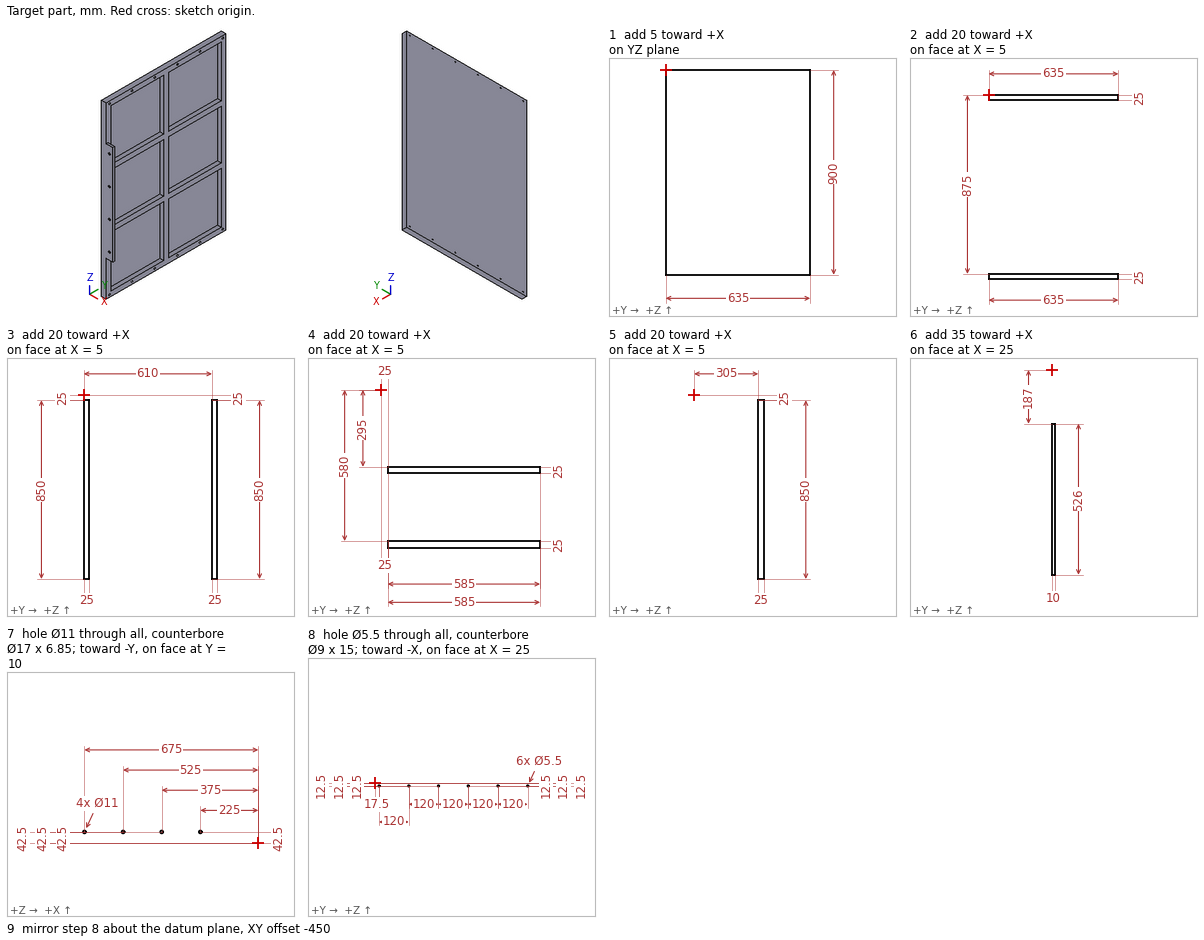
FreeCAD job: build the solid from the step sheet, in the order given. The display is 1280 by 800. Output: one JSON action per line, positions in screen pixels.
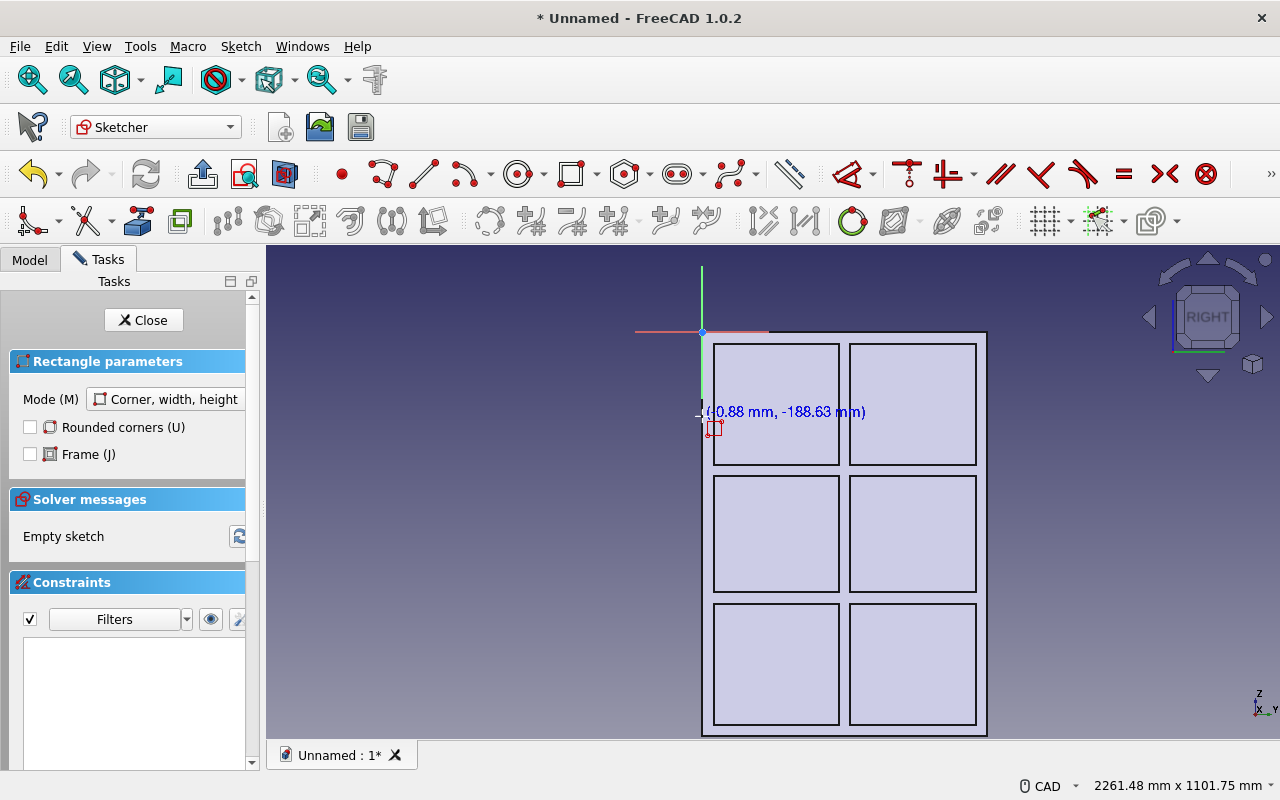
{"action": "left_click", "coordinate": [702, 416]}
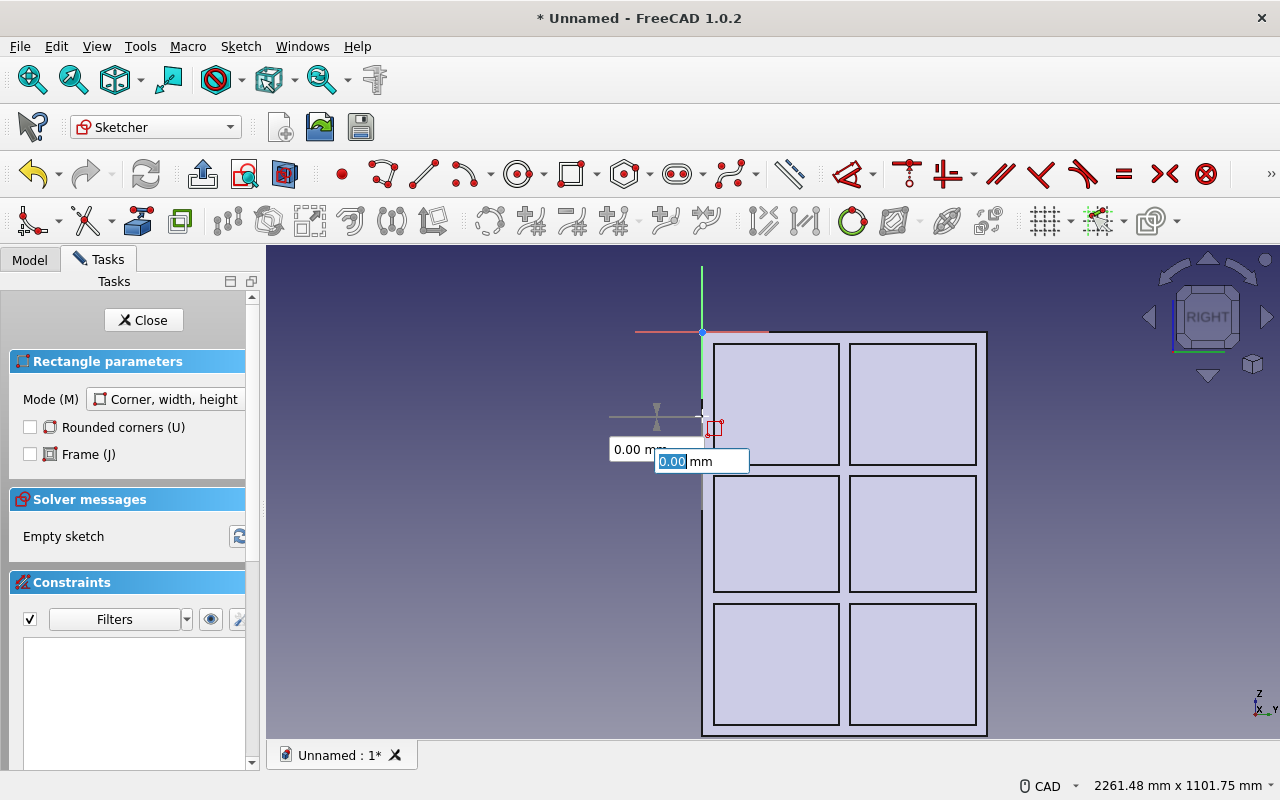
{"action": "scroll", "coordinate": [707, 652], "scroll_direction": "up", "scroll_amount": 7}
{"action": "mouse_move", "coordinate": [705, 650]}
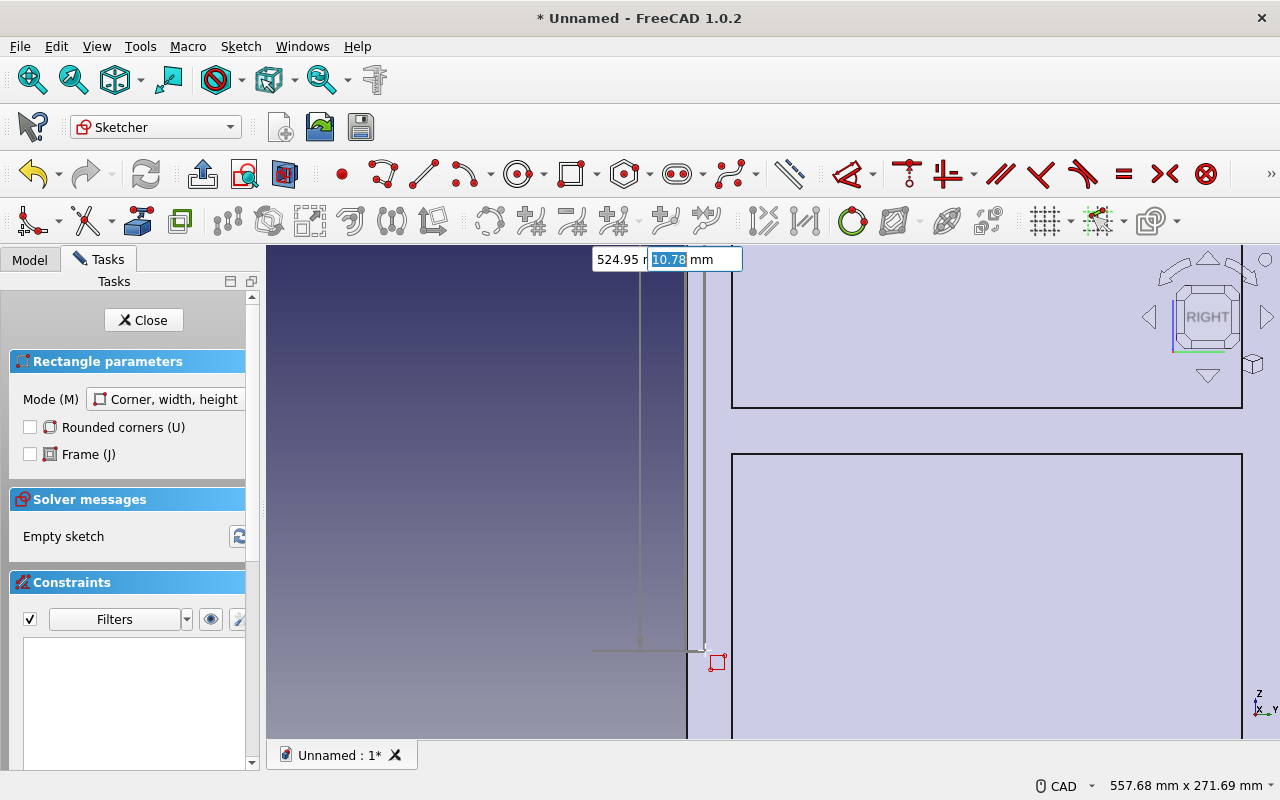
{"action": "type", "text": "10"}
{"action": "key", "text": "Tab"}
{"action": "type", "text": "526"}
{"action": "key", "text": "Return"}
{"action": "key", "text": "Escape"}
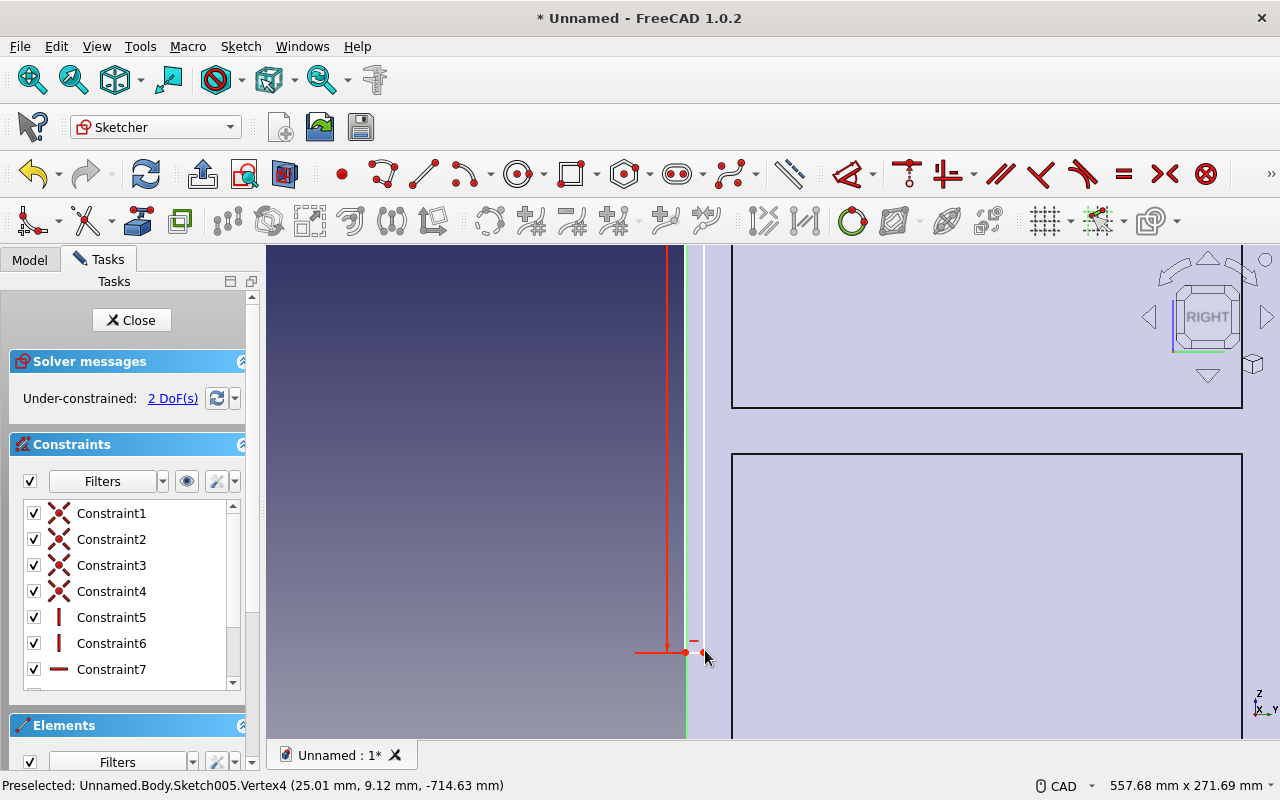
{"action": "scroll", "coordinate": [707, 652], "scroll_direction": "down", "scroll_amount": 7}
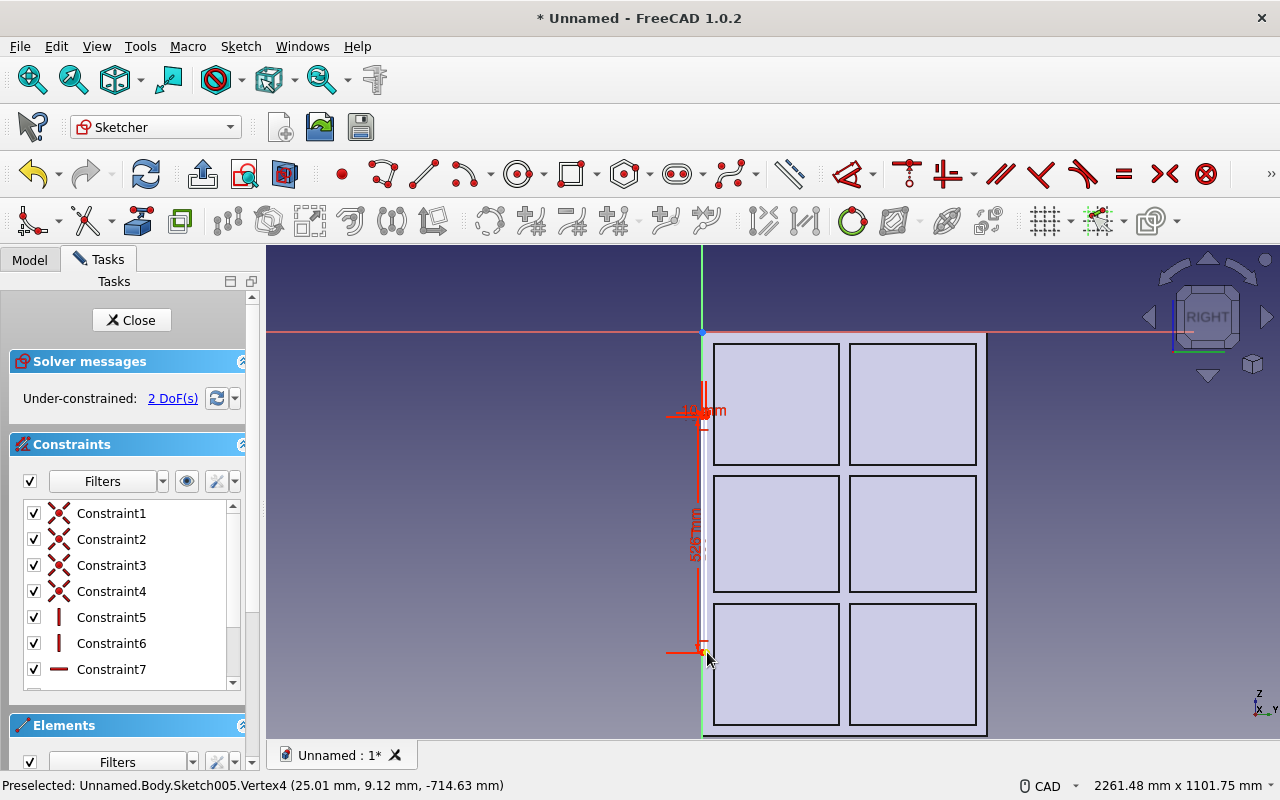
{"action": "scroll", "coordinate": [702, 417], "scroll_direction": "up", "scroll_amount": 6}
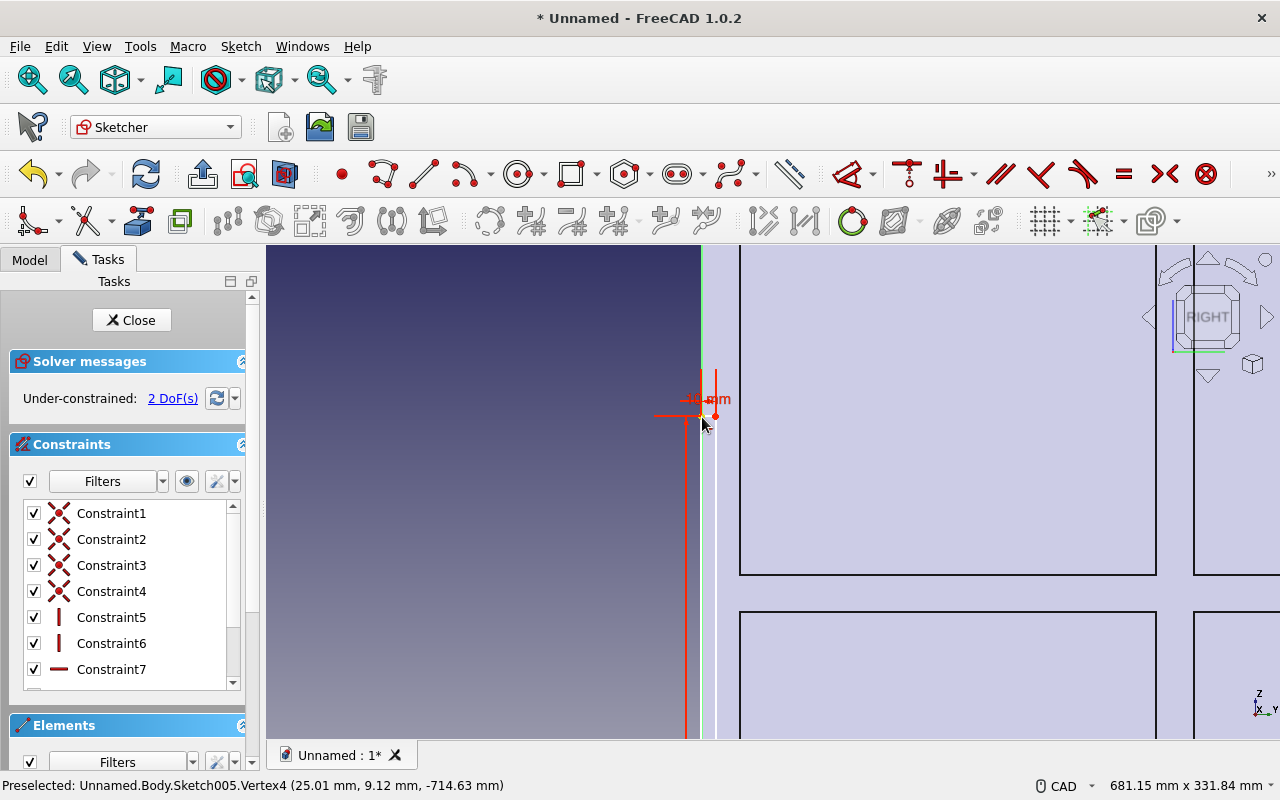
{"action": "left_click", "coordinate": [701, 416]}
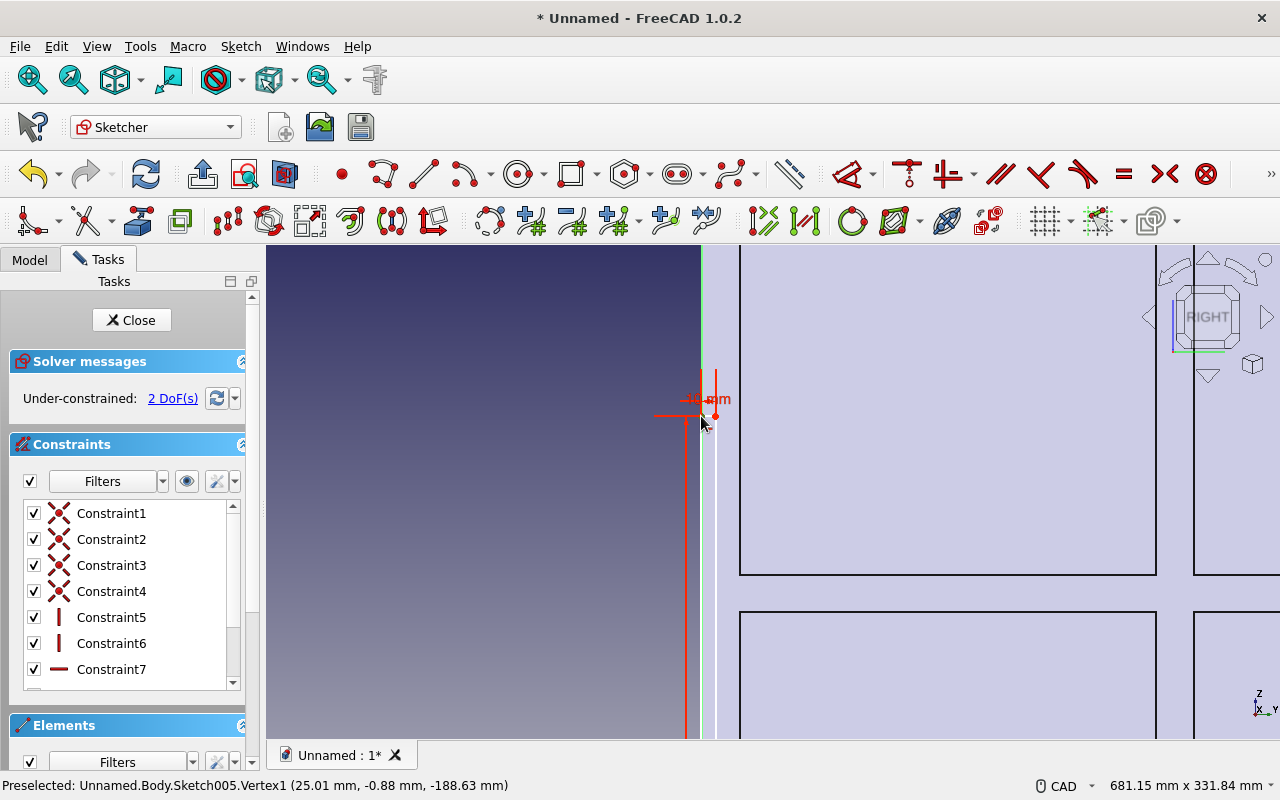
{"action": "left_click", "coordinate": [702, 367]}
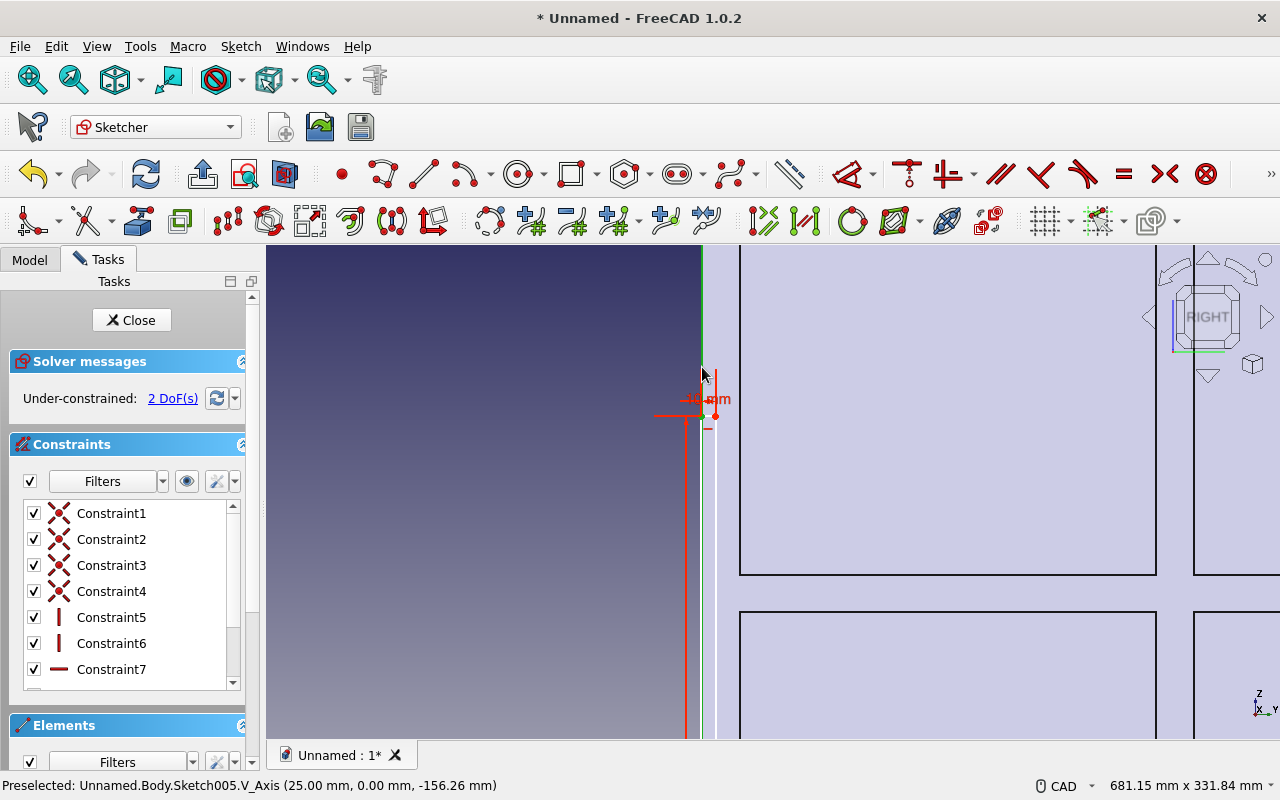
{"action": "left_click", "coordinate": [907, 174]}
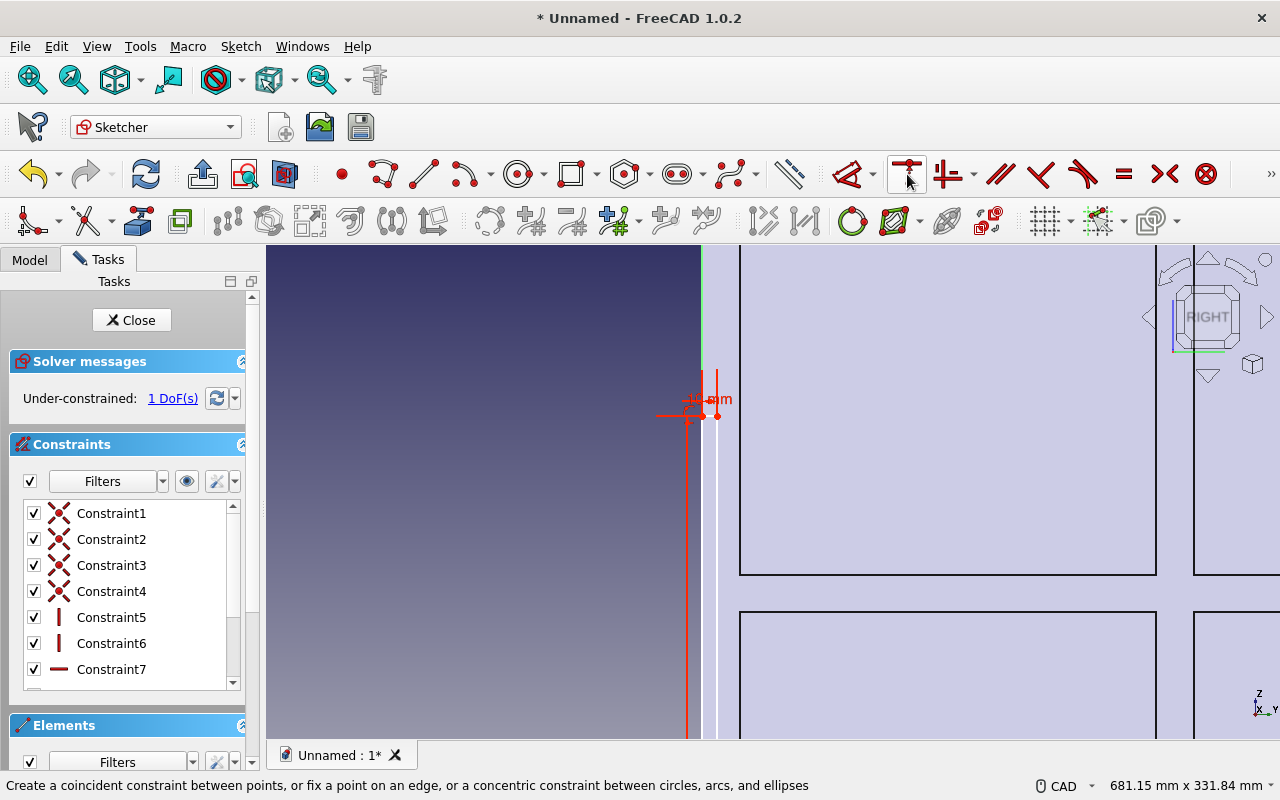
{"action": "left_click", "coordinate": [846, 174]}